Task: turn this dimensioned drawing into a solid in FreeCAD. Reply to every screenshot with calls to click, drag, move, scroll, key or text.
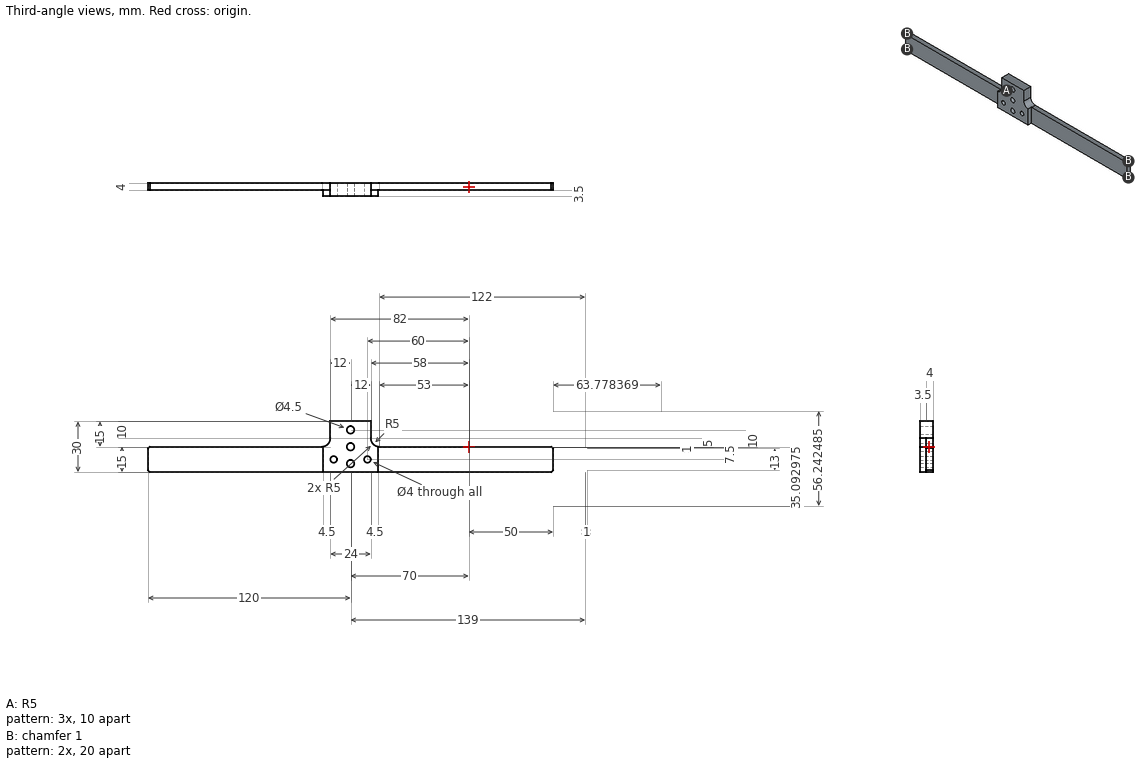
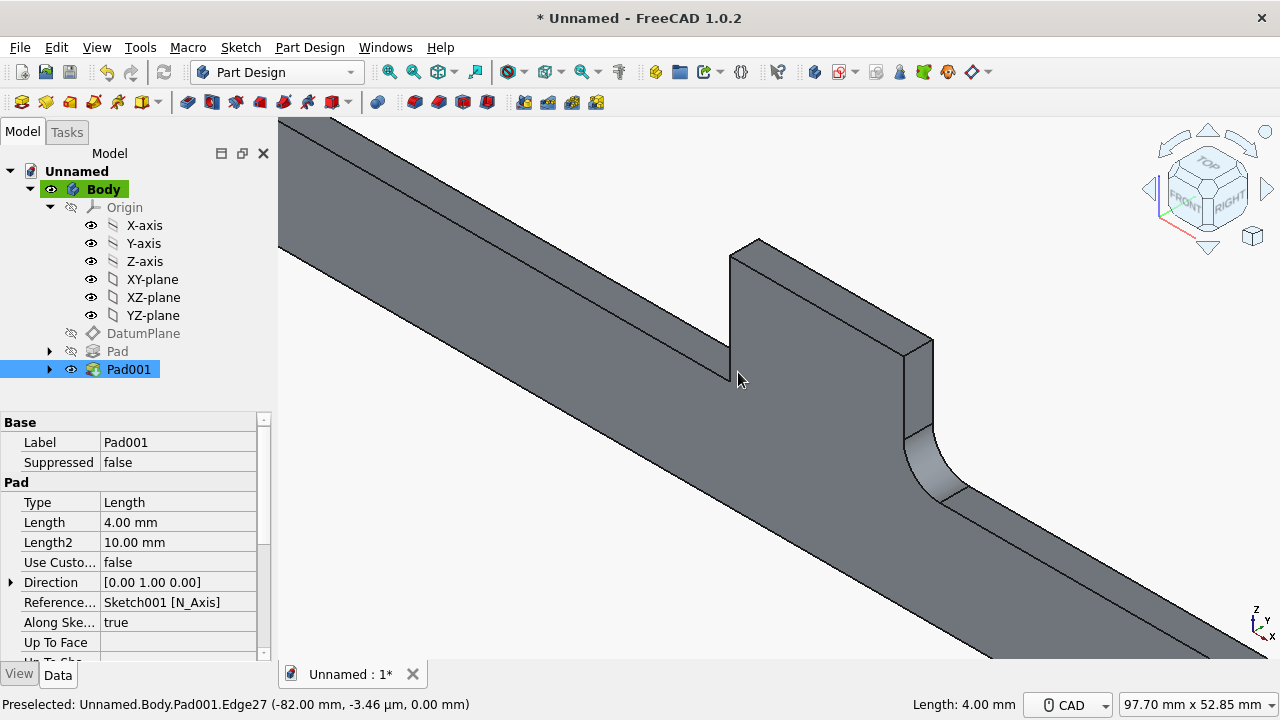
click(416, 102)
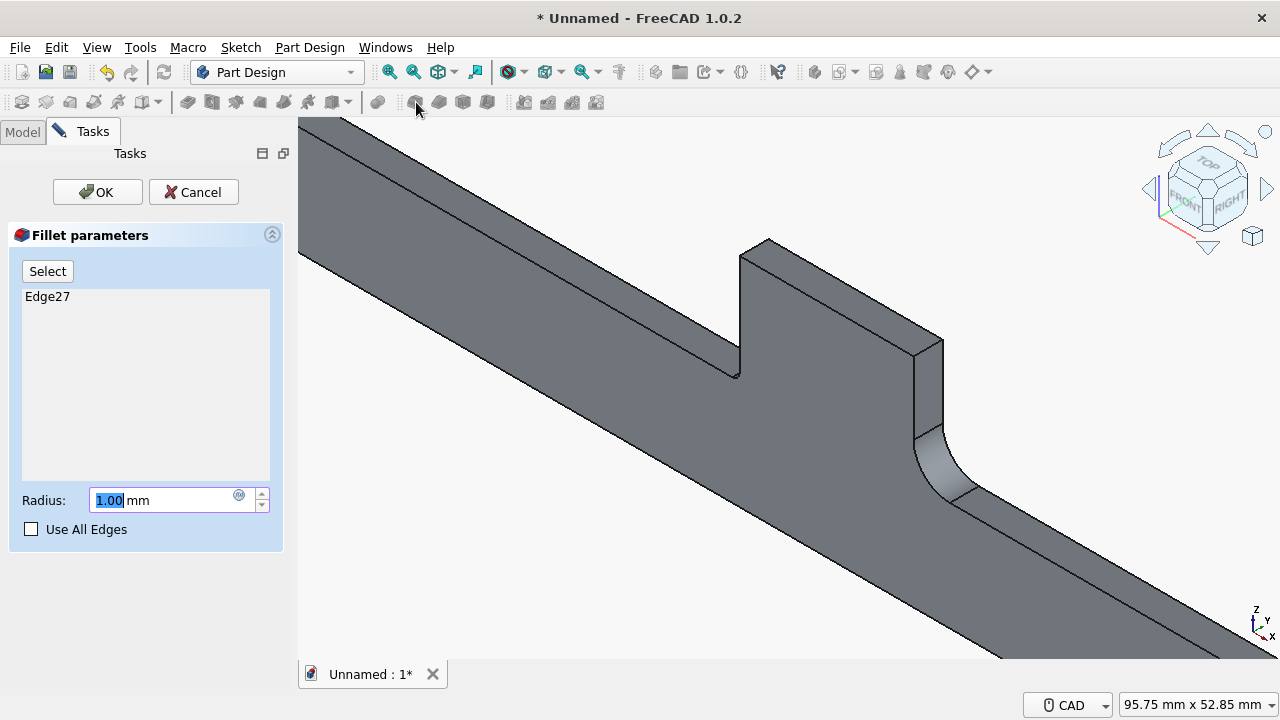
text(5)
key(Tab)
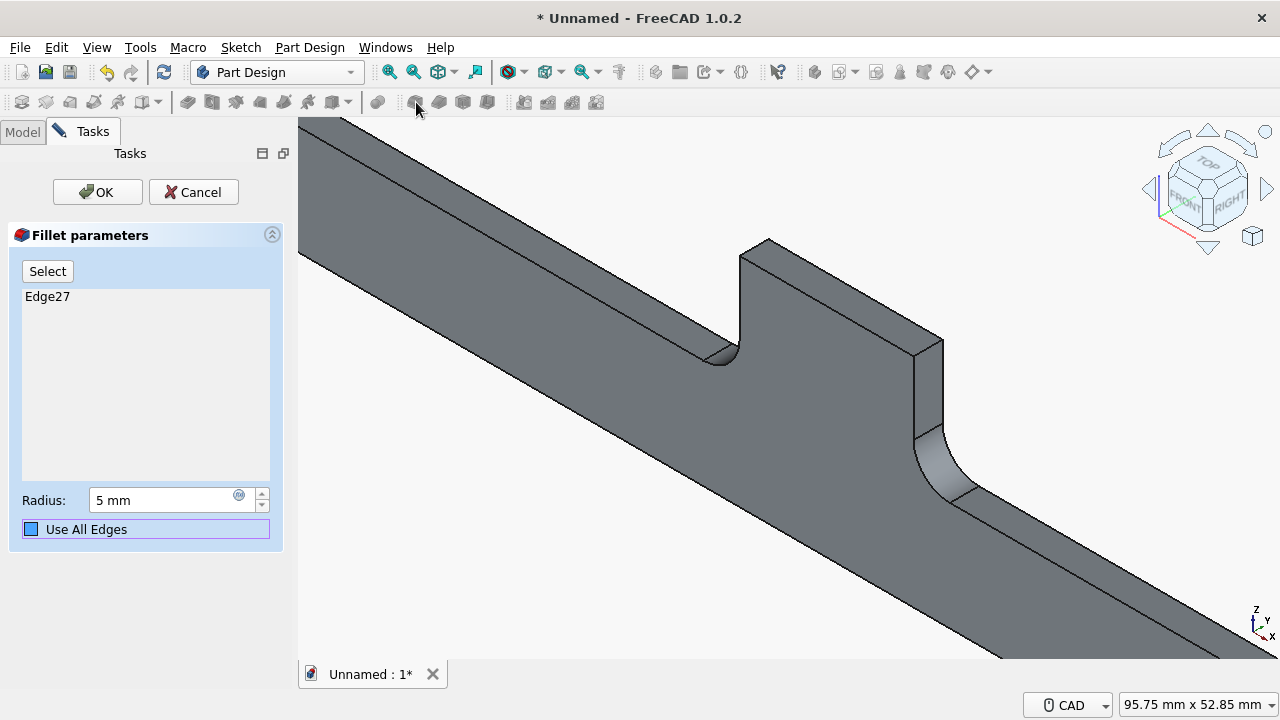
click(98, 192)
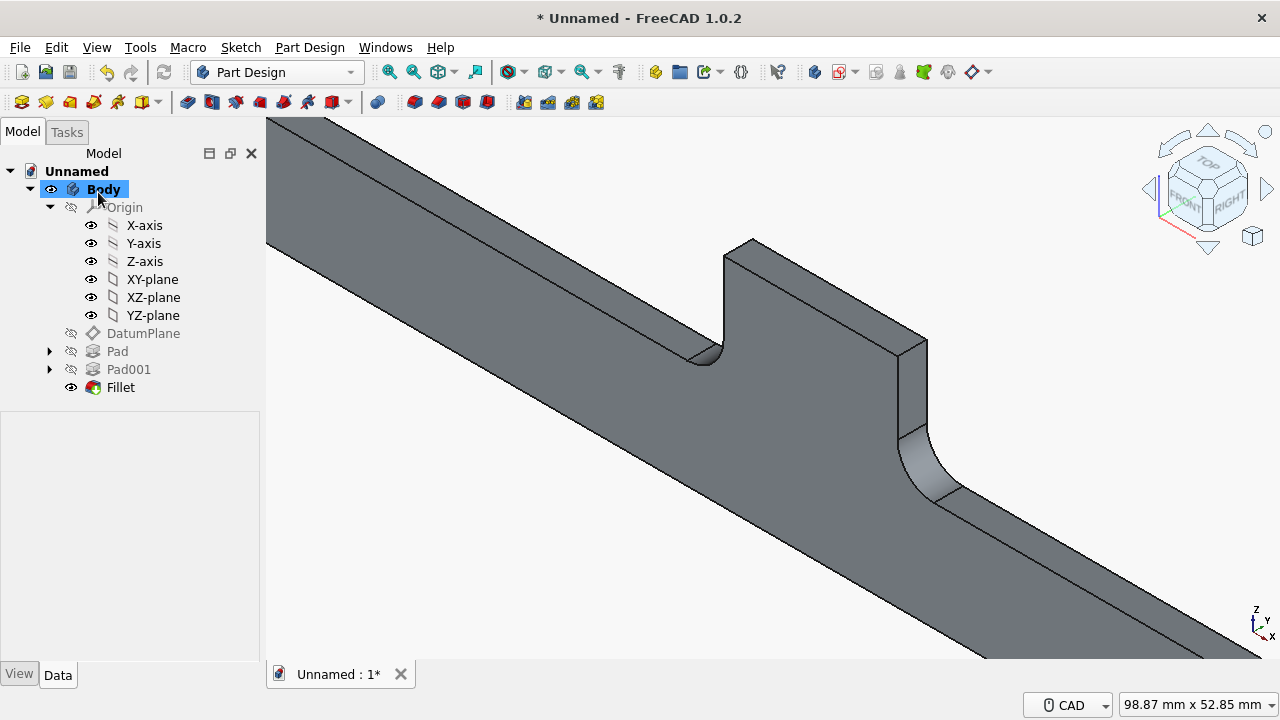
click(390, 72)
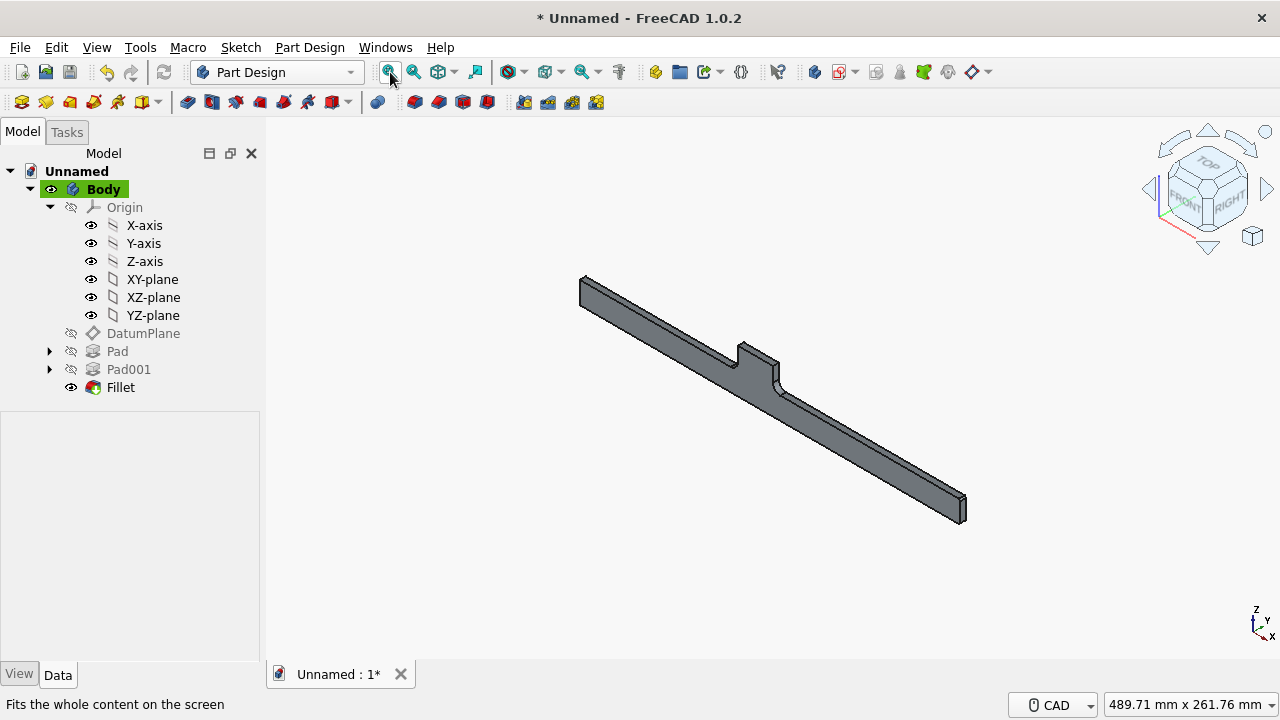
click(933, 497)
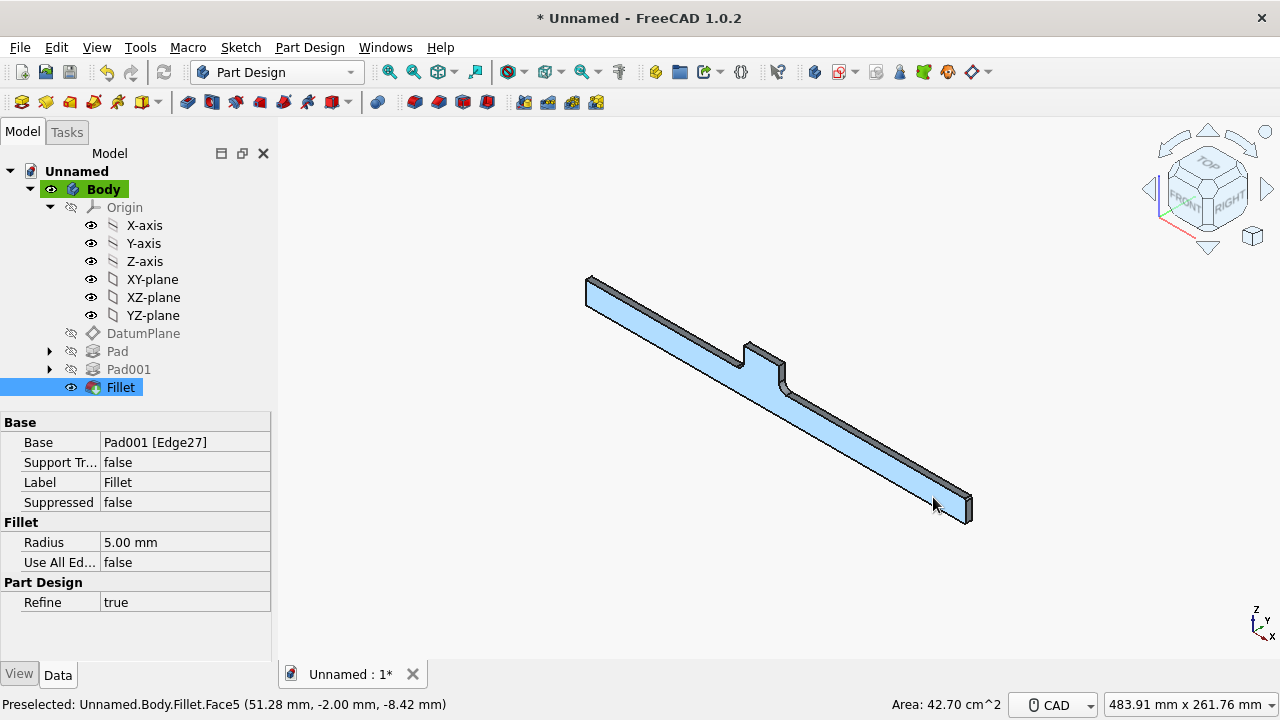
click(840, 72)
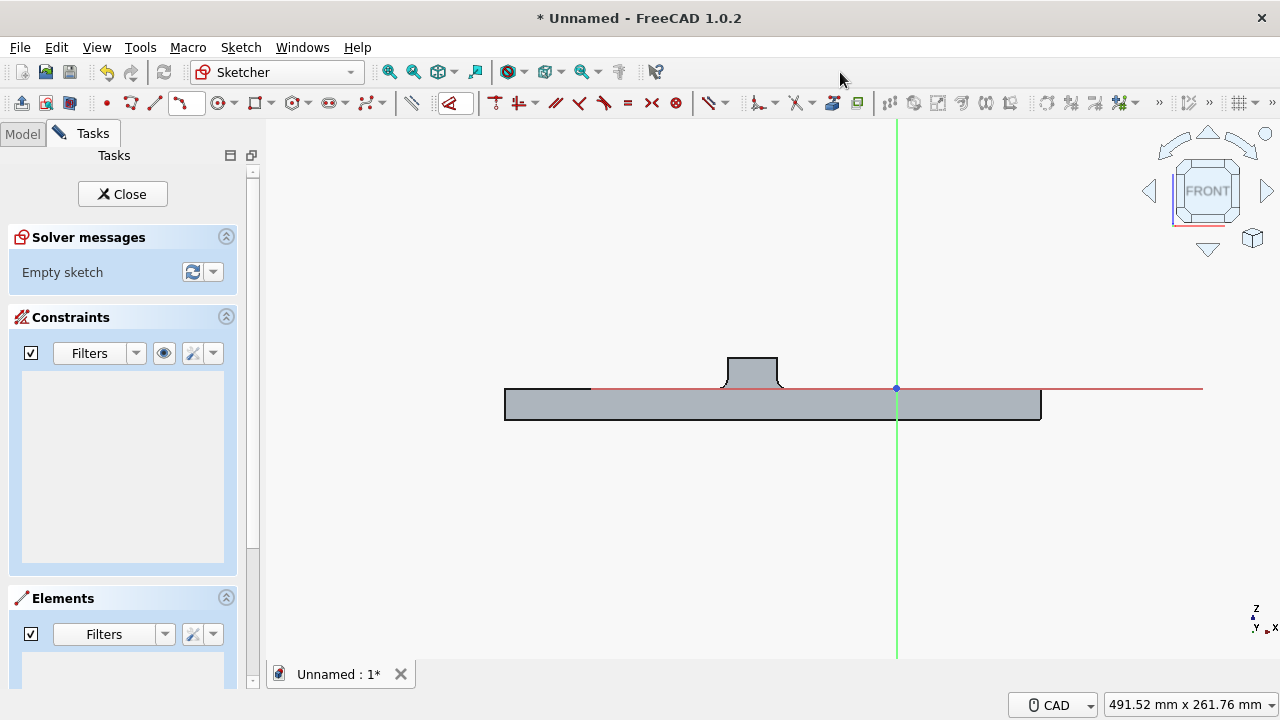
scroll(762, 389, up, 9)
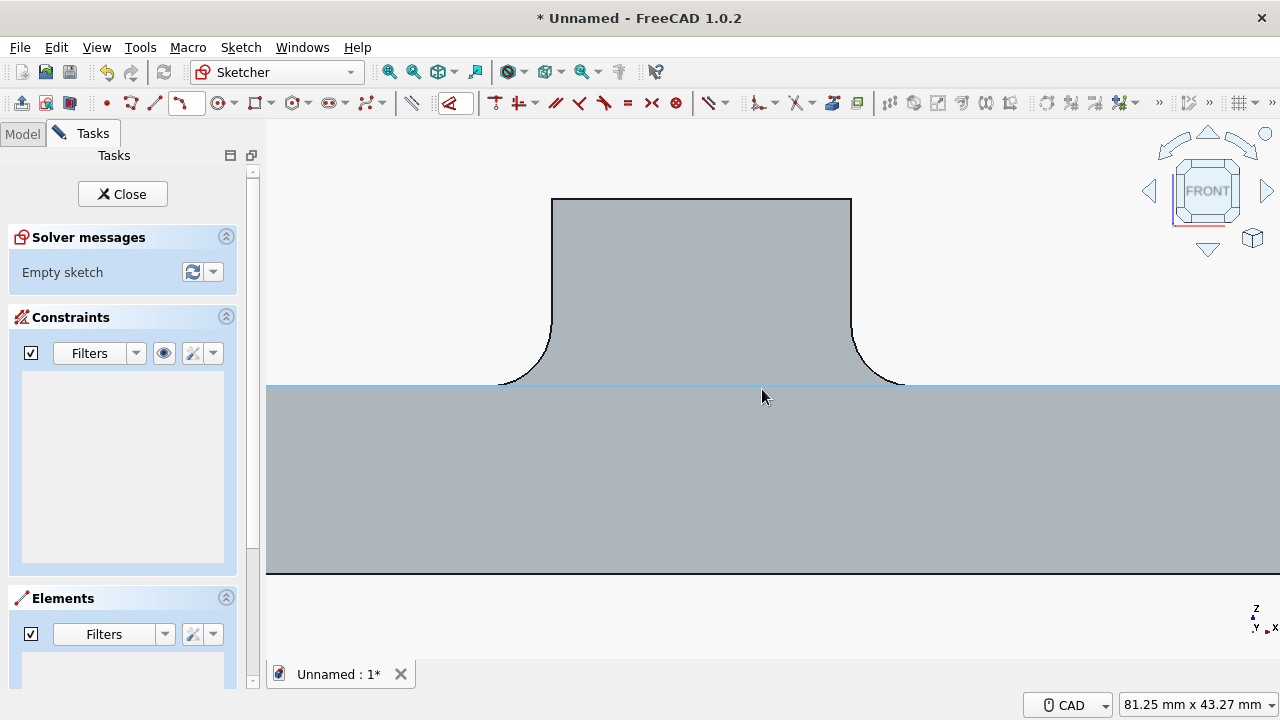
click(256, 104)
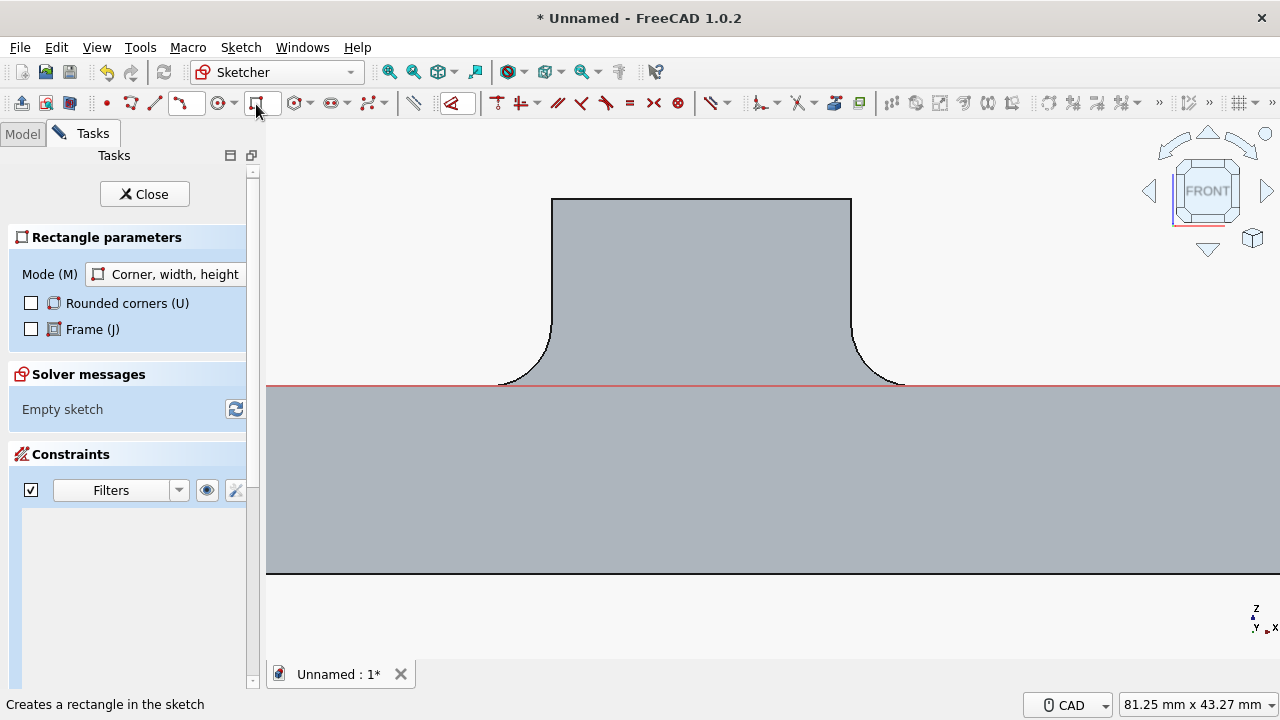
click(552, 199)
click(851, 574)
key(Escape)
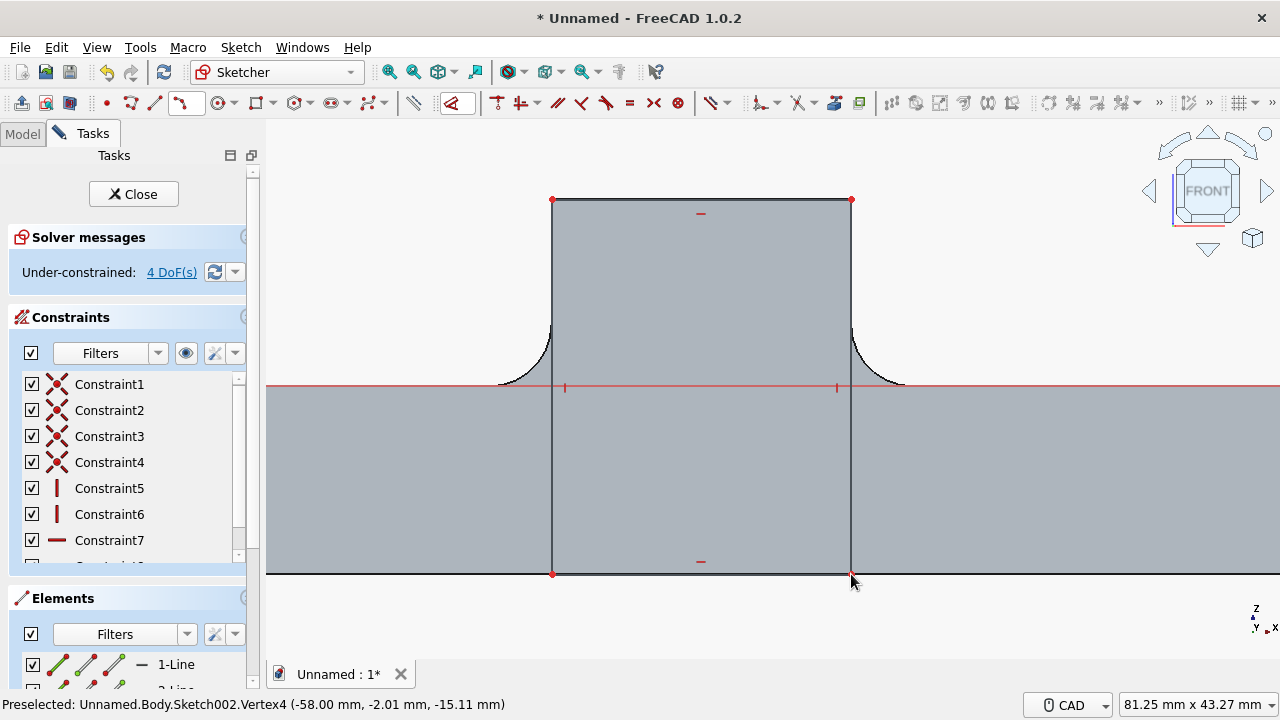
click(552, 312)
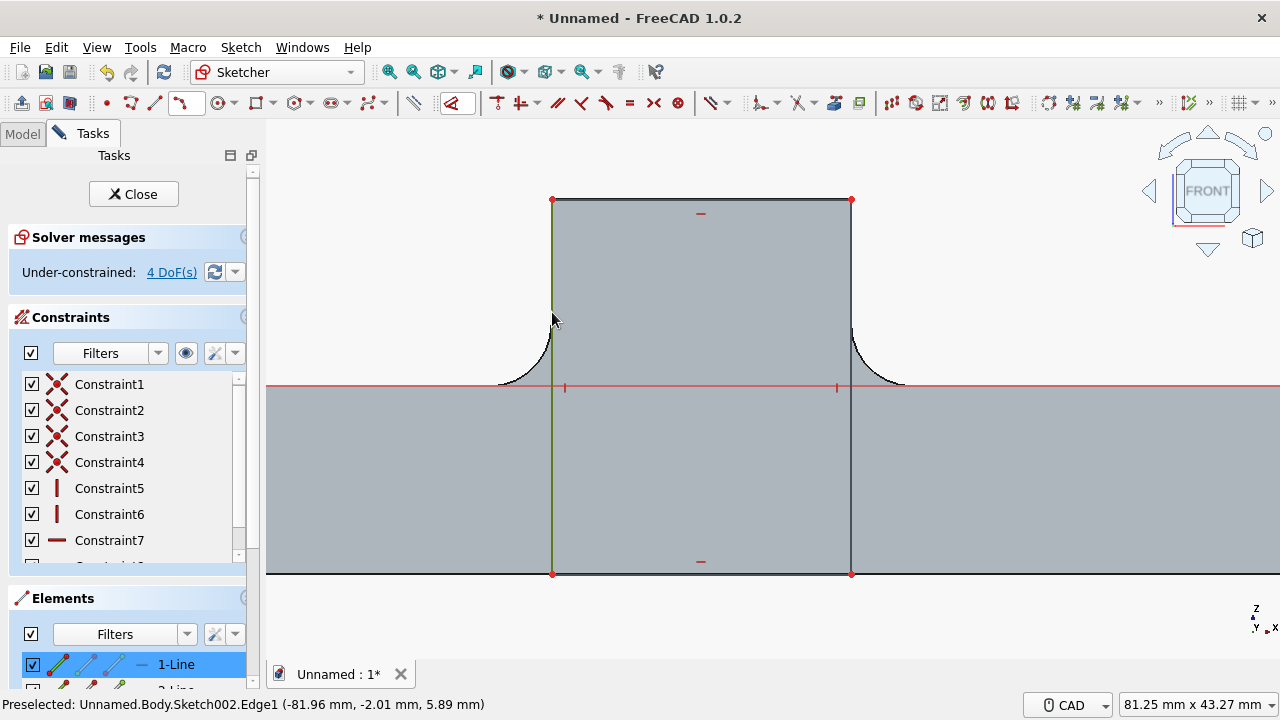
click(470, 104)